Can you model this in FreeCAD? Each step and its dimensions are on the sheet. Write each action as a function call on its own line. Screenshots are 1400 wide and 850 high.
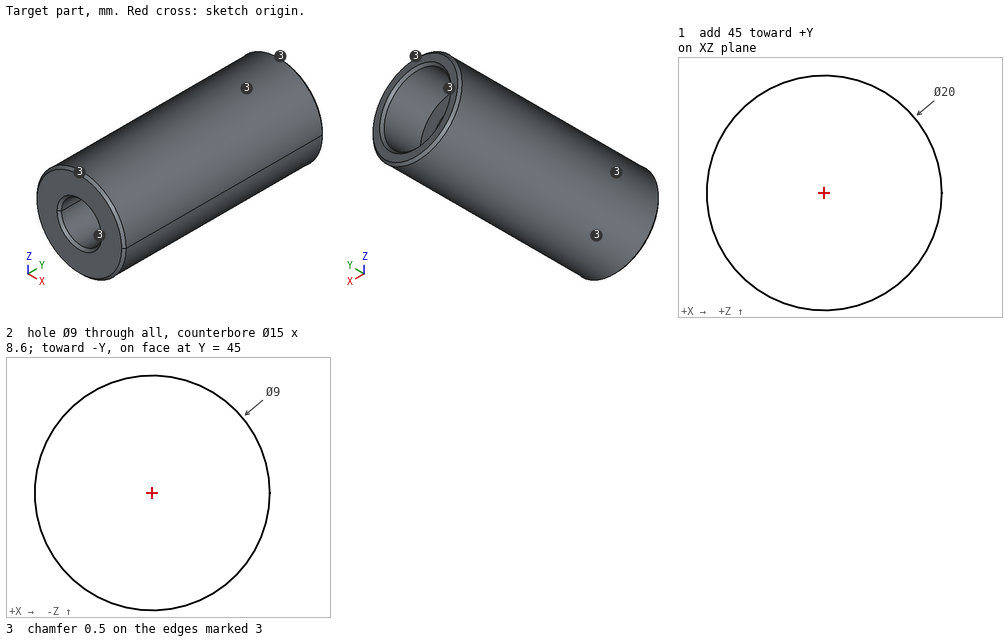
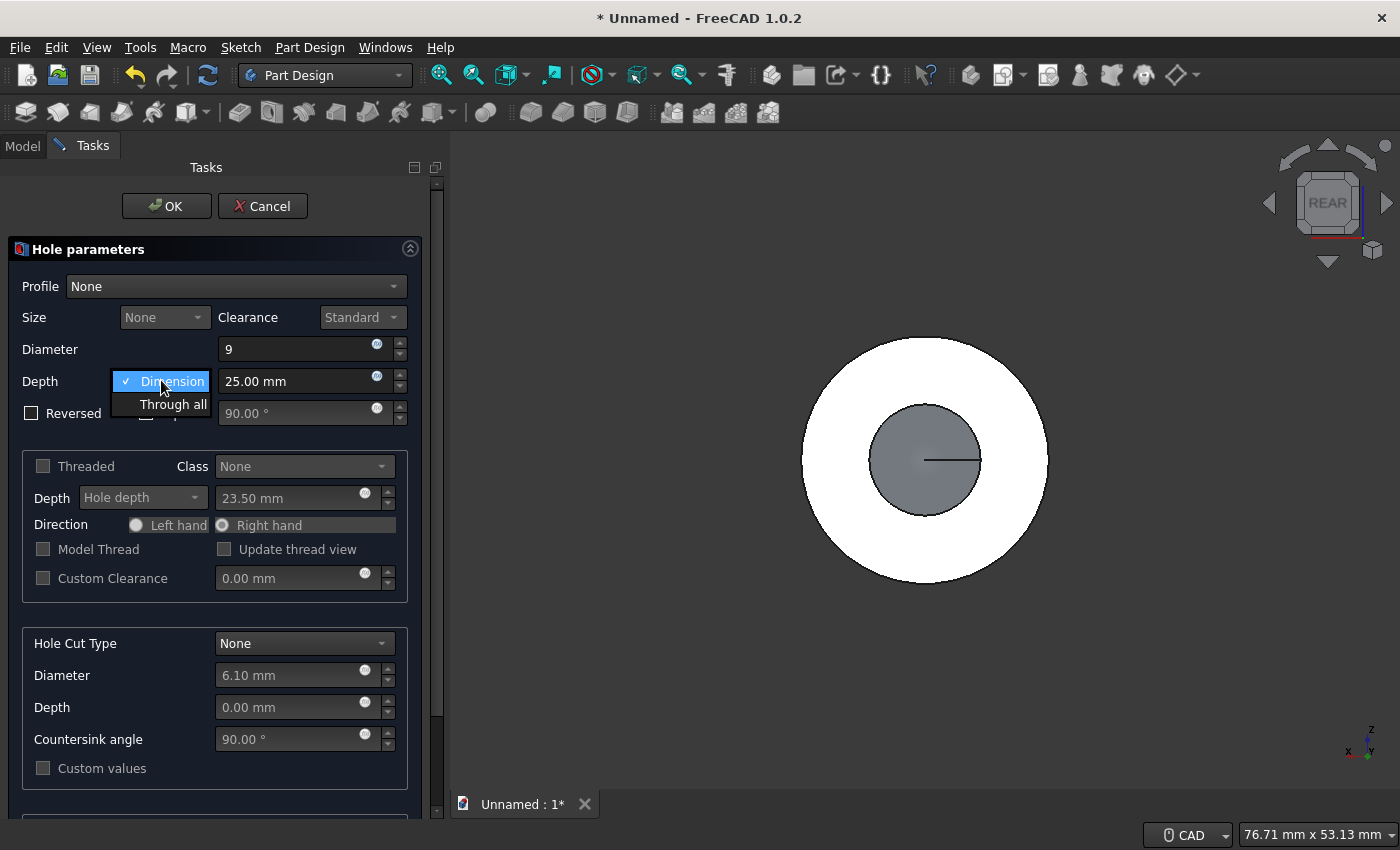
click(160, 404)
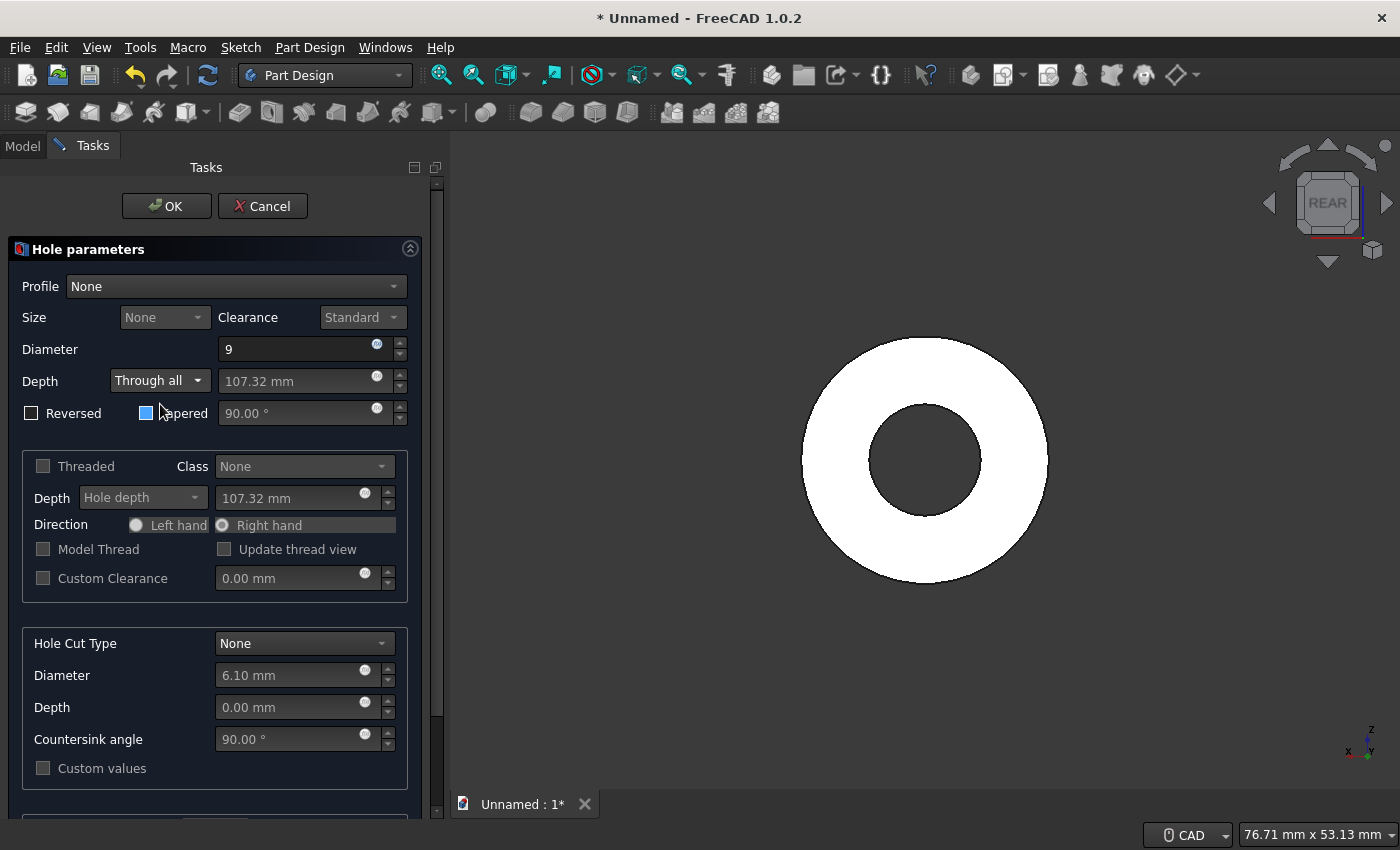
click(306, 644)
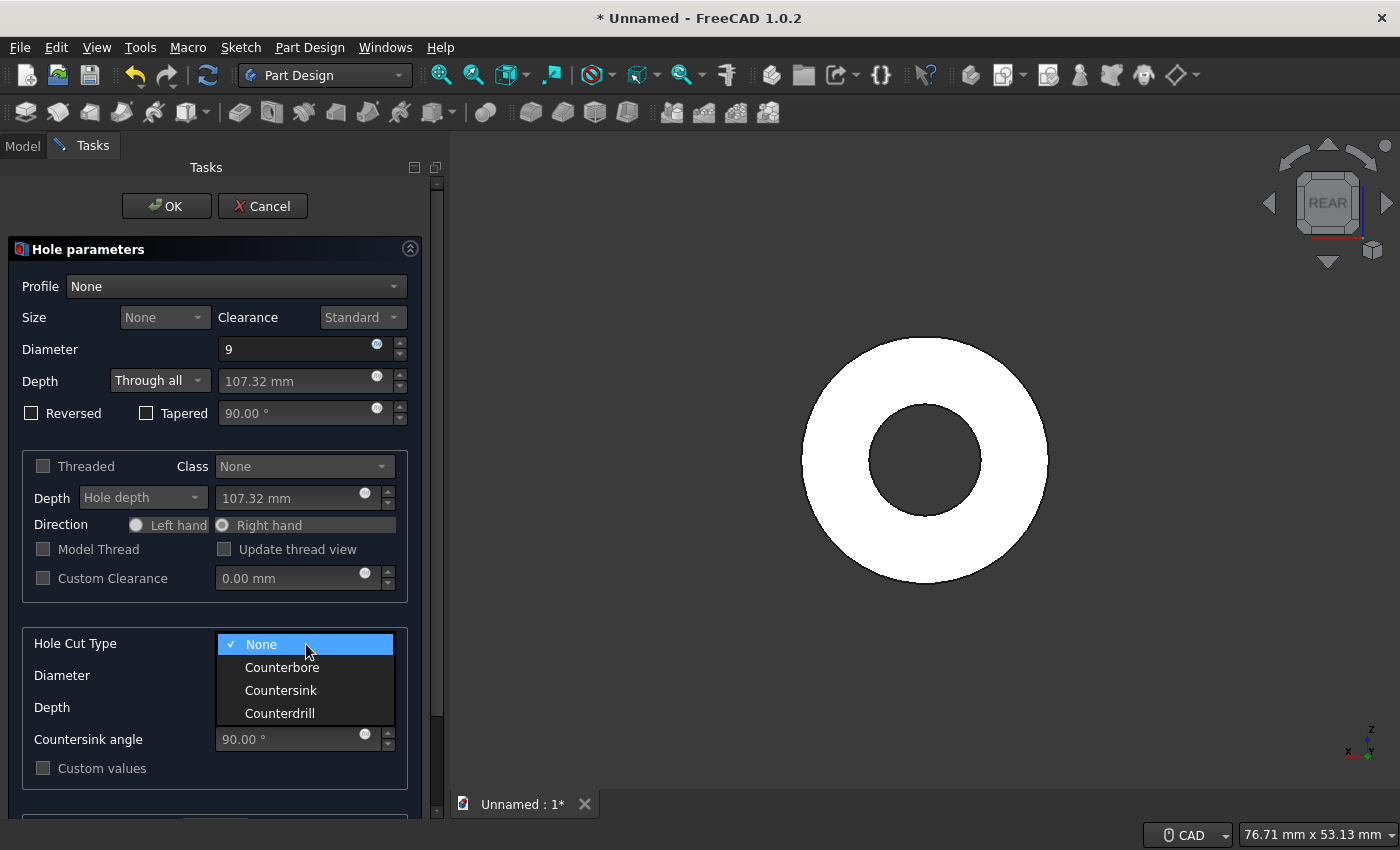
click(304, 668)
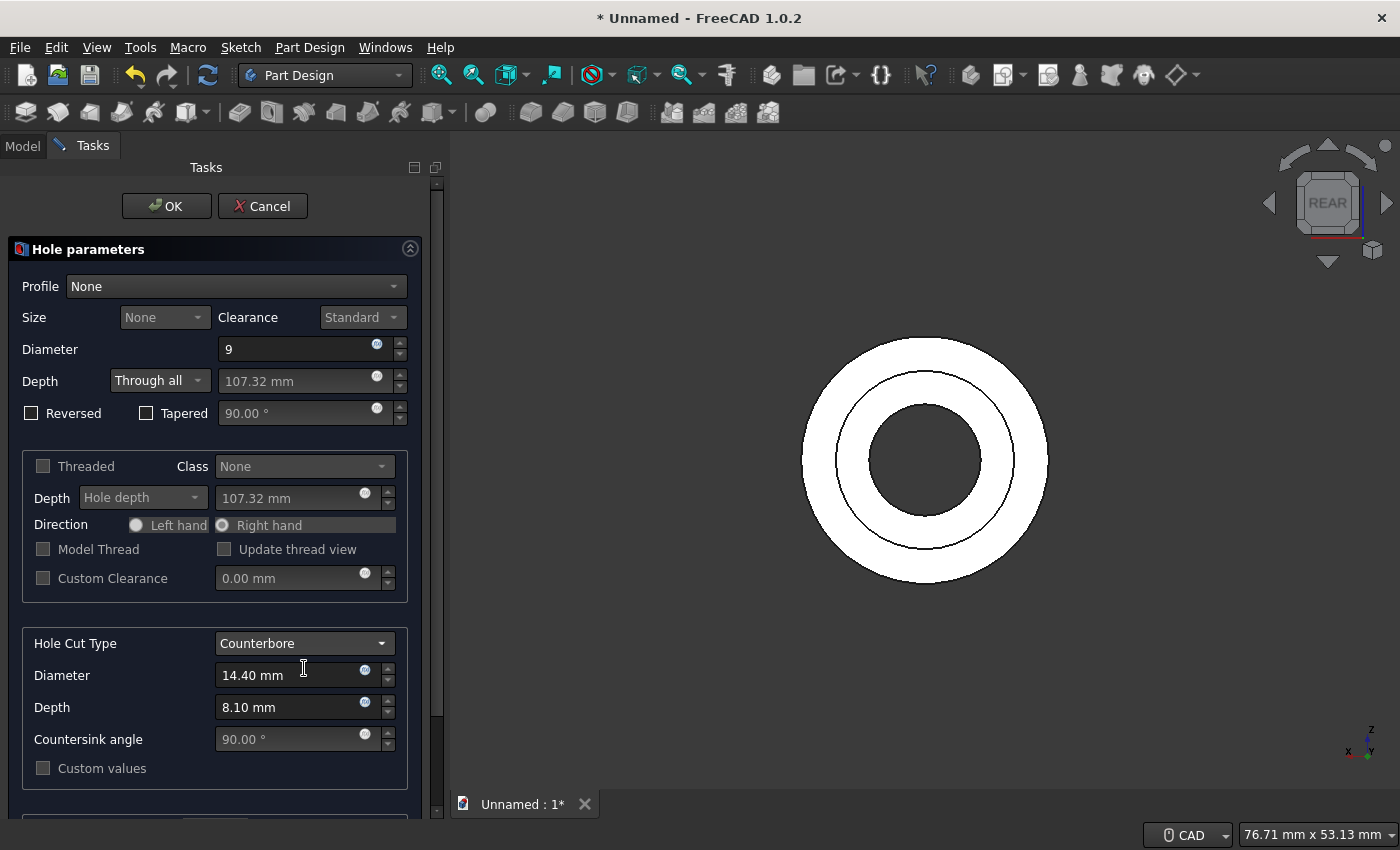
triple_click(298, 675)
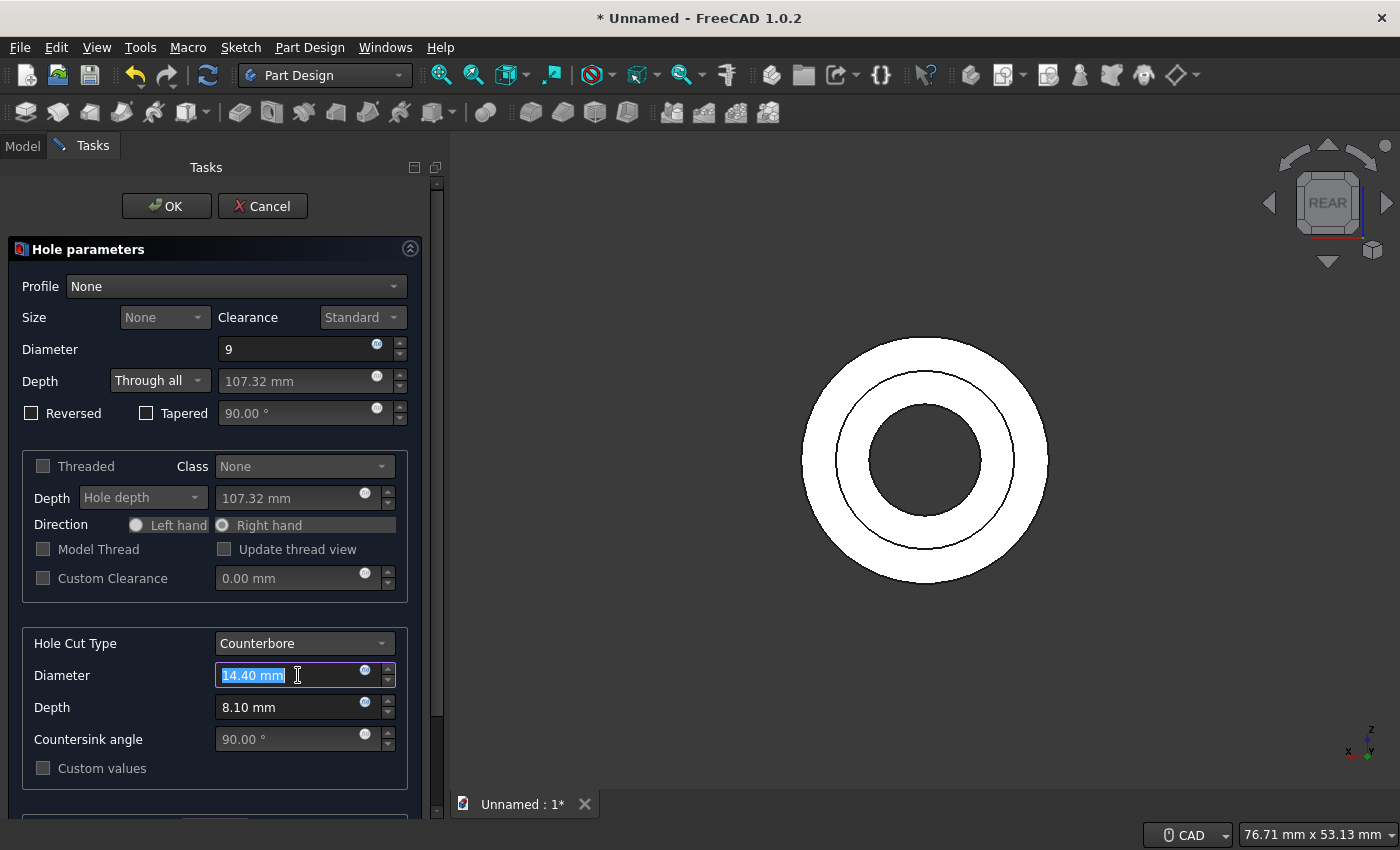
text(15)
key(Tab)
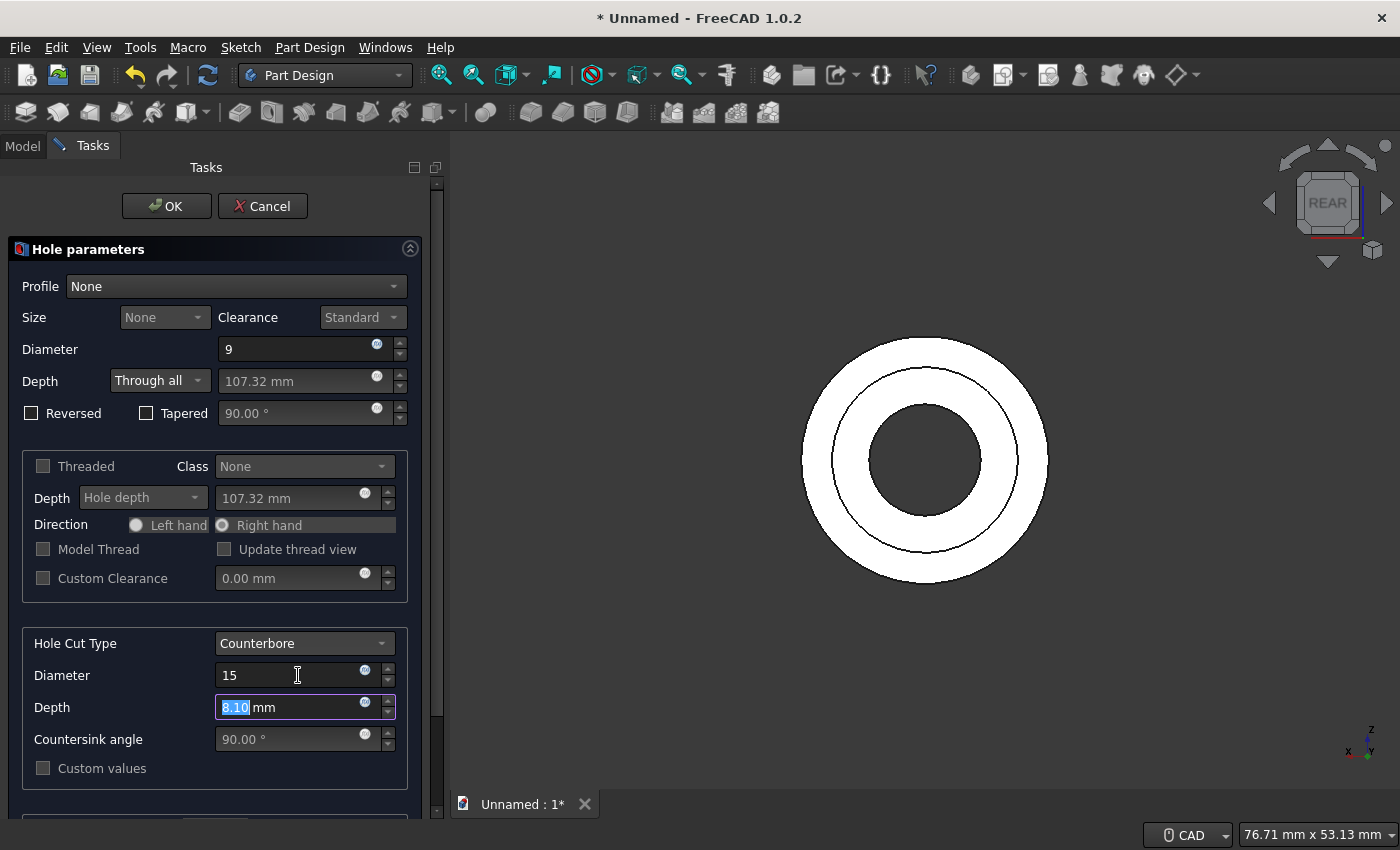
text(8.6)
key(Tab)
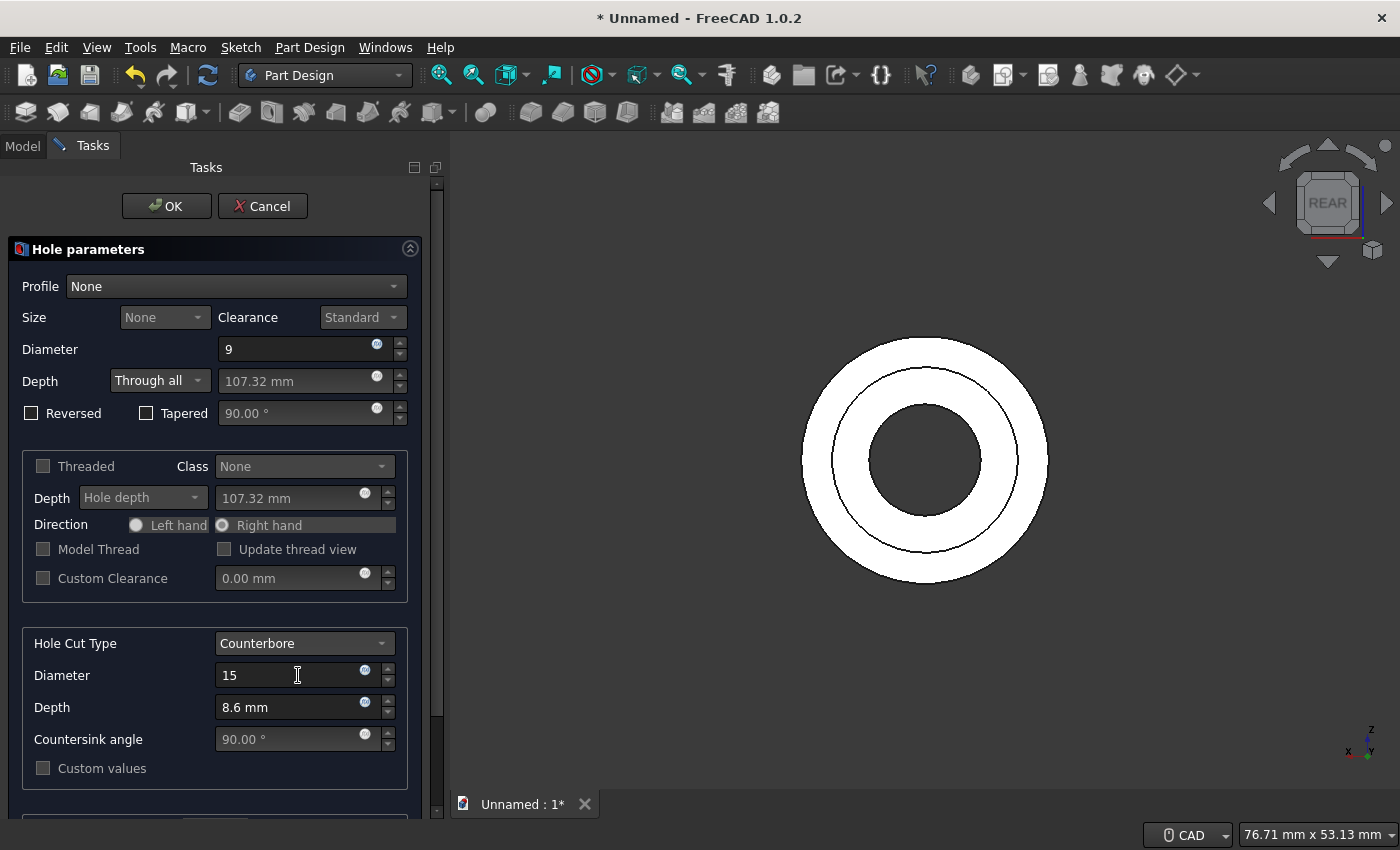
click(167, 206)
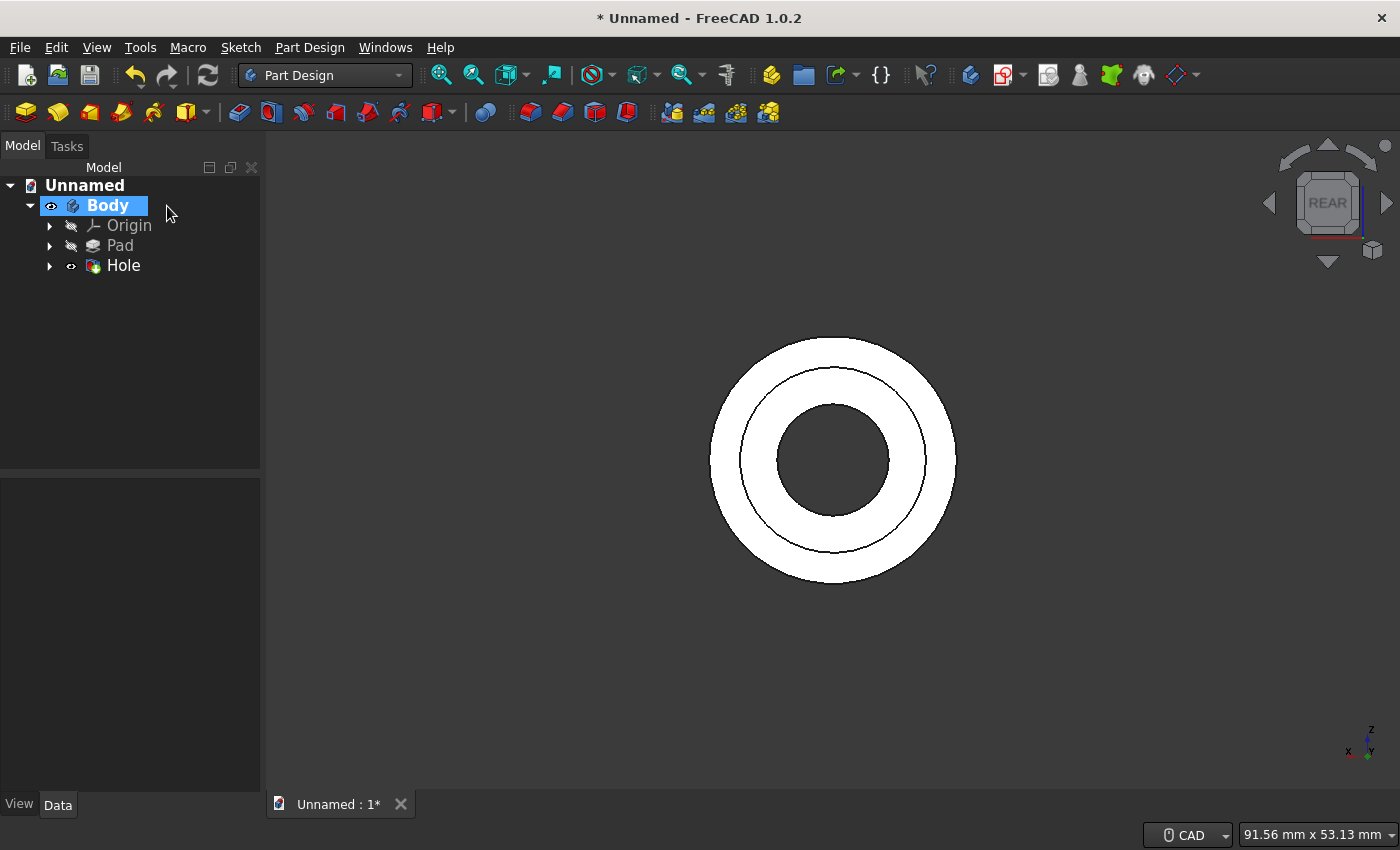
click(442, 76)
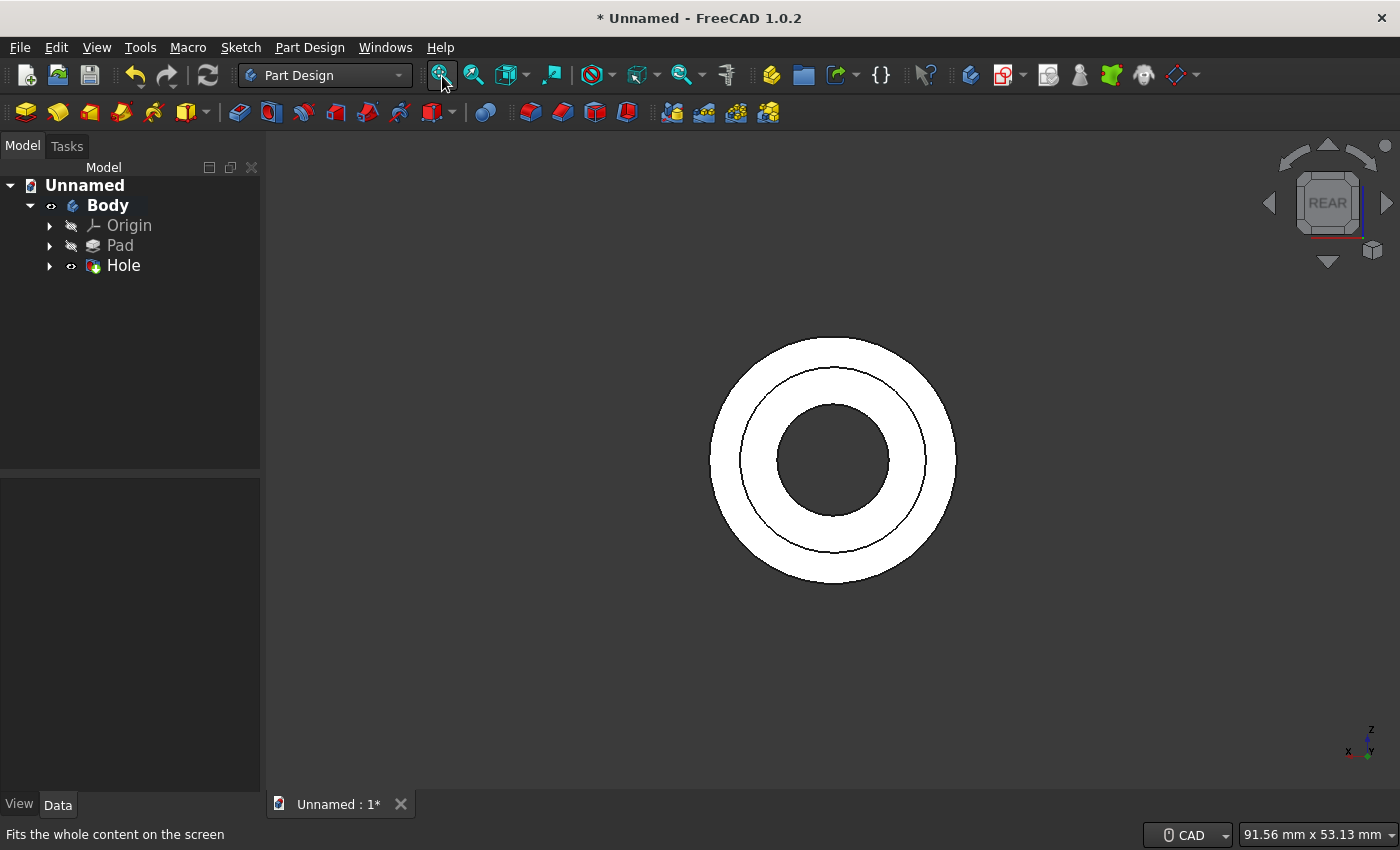
click(957, 459)